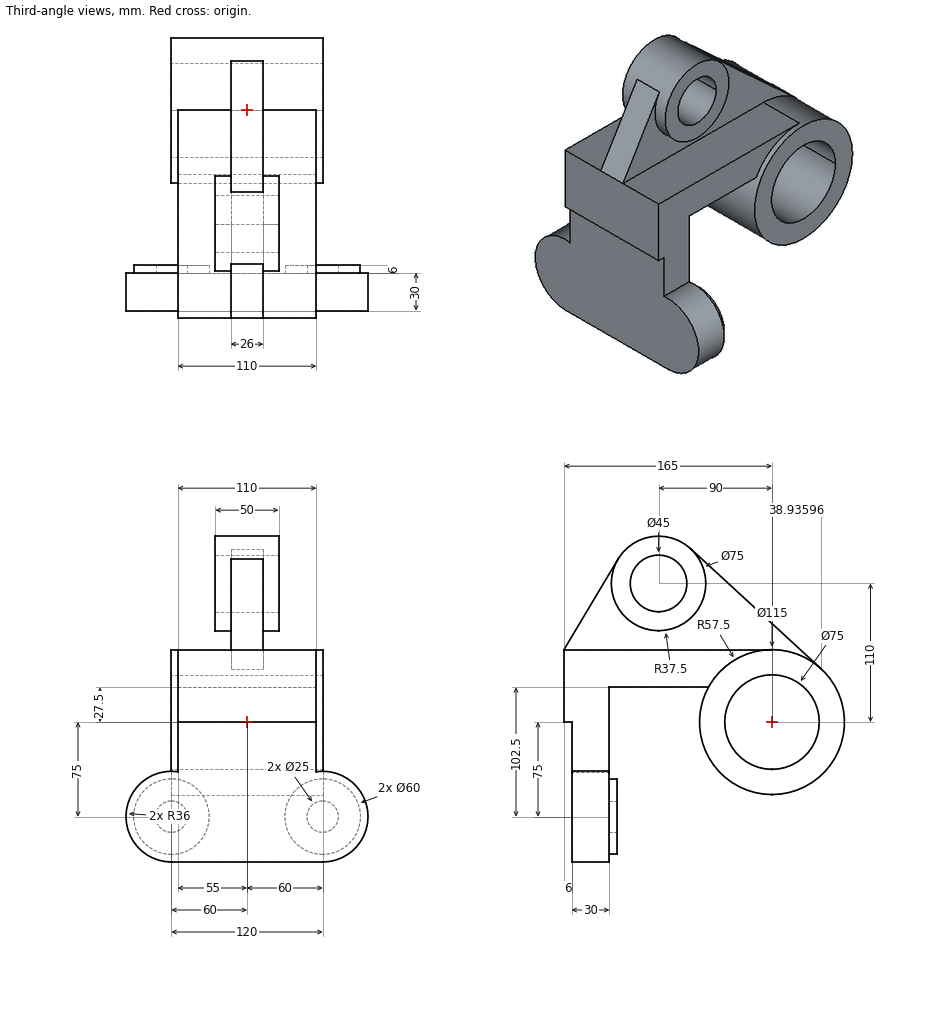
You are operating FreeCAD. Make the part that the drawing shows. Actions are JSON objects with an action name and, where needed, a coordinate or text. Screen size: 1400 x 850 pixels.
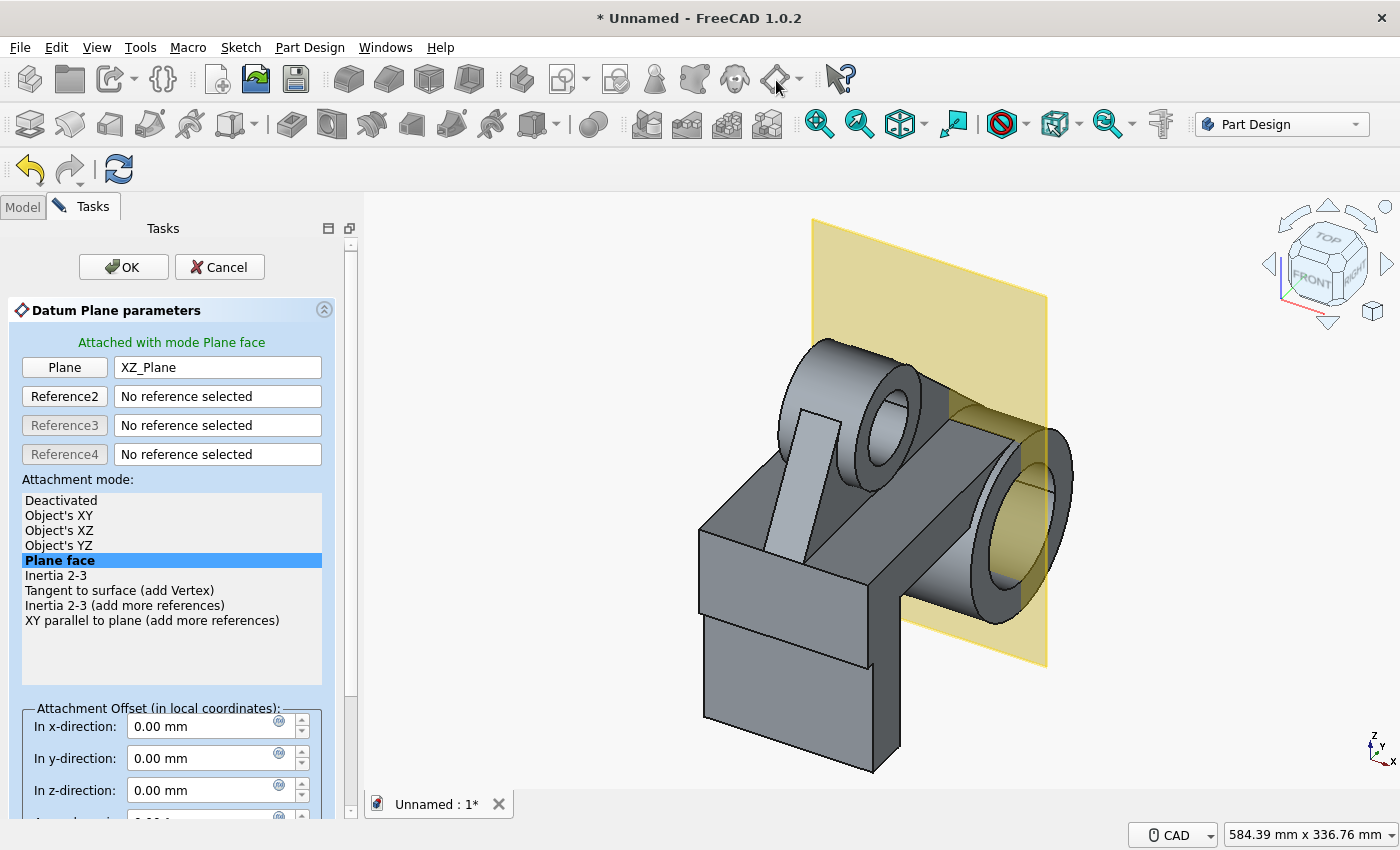
{"action": "triple_click", "coordinate": [210, 790]}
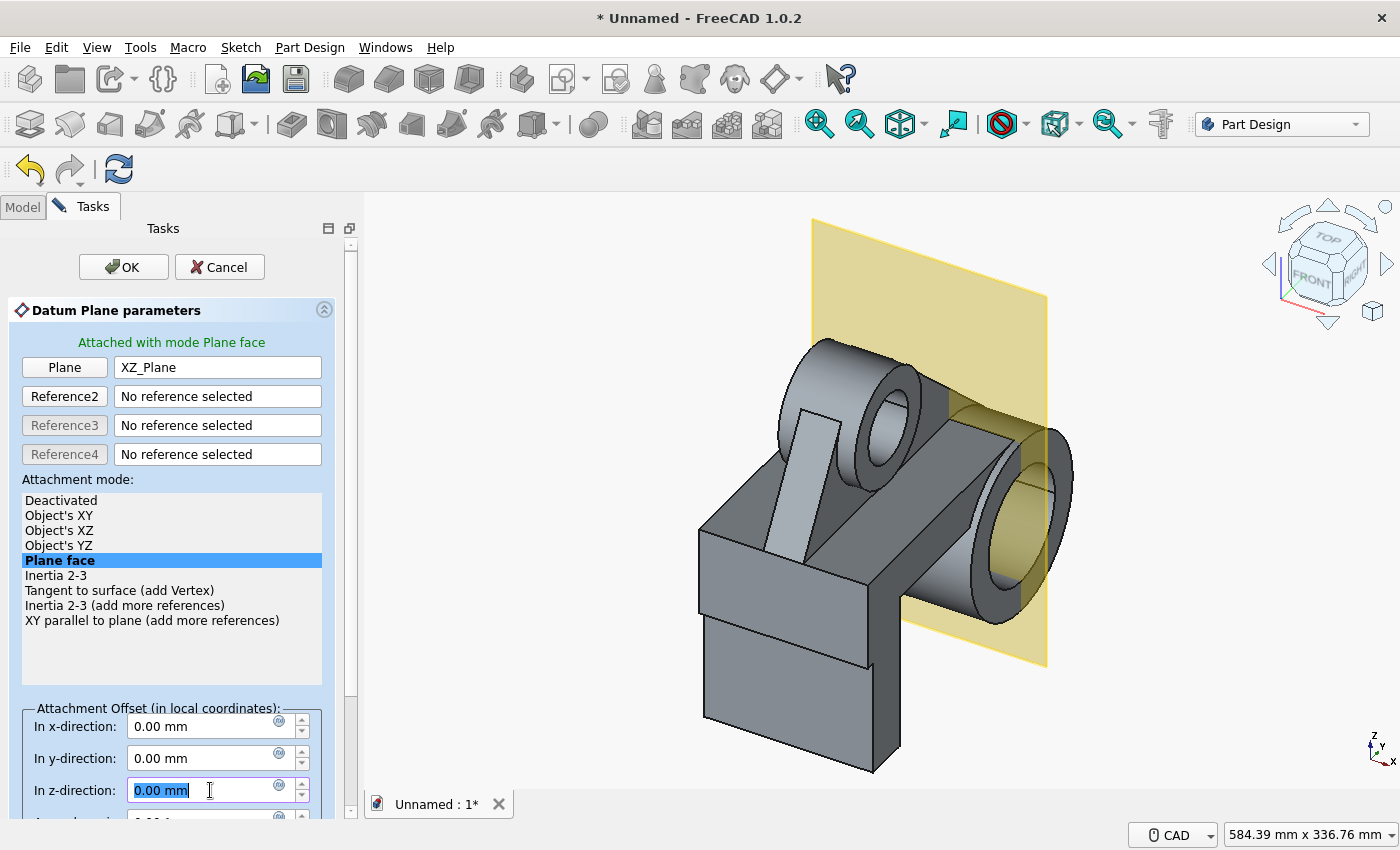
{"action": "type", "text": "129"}
{"action": "key", "text": "Tab"}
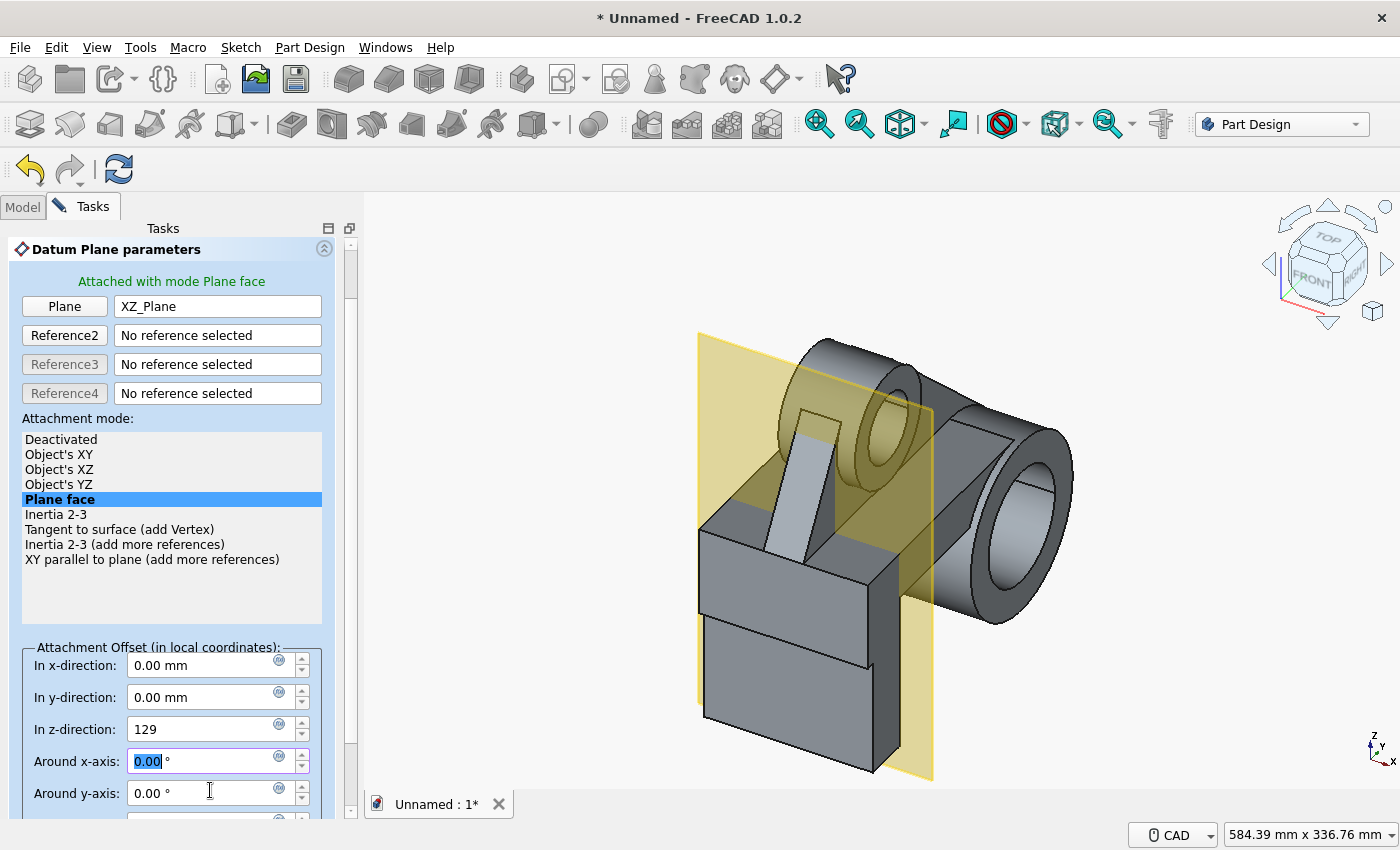
{"action": "scroll", "coordinate": [351, 528], "scroll_direction": "up", "scroll_amount": 2}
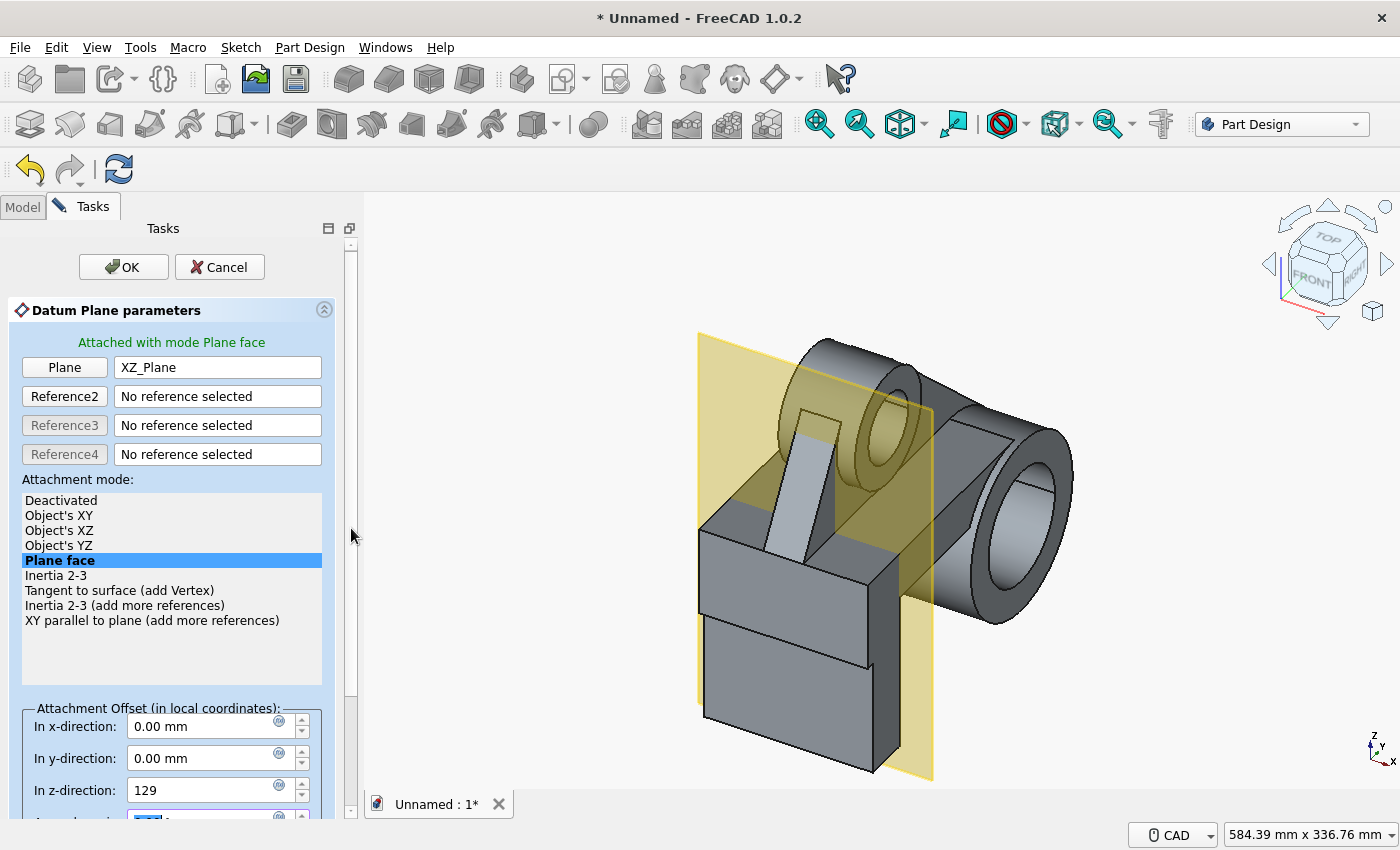
{"action": "left_click", "coordinate": [124, 267]}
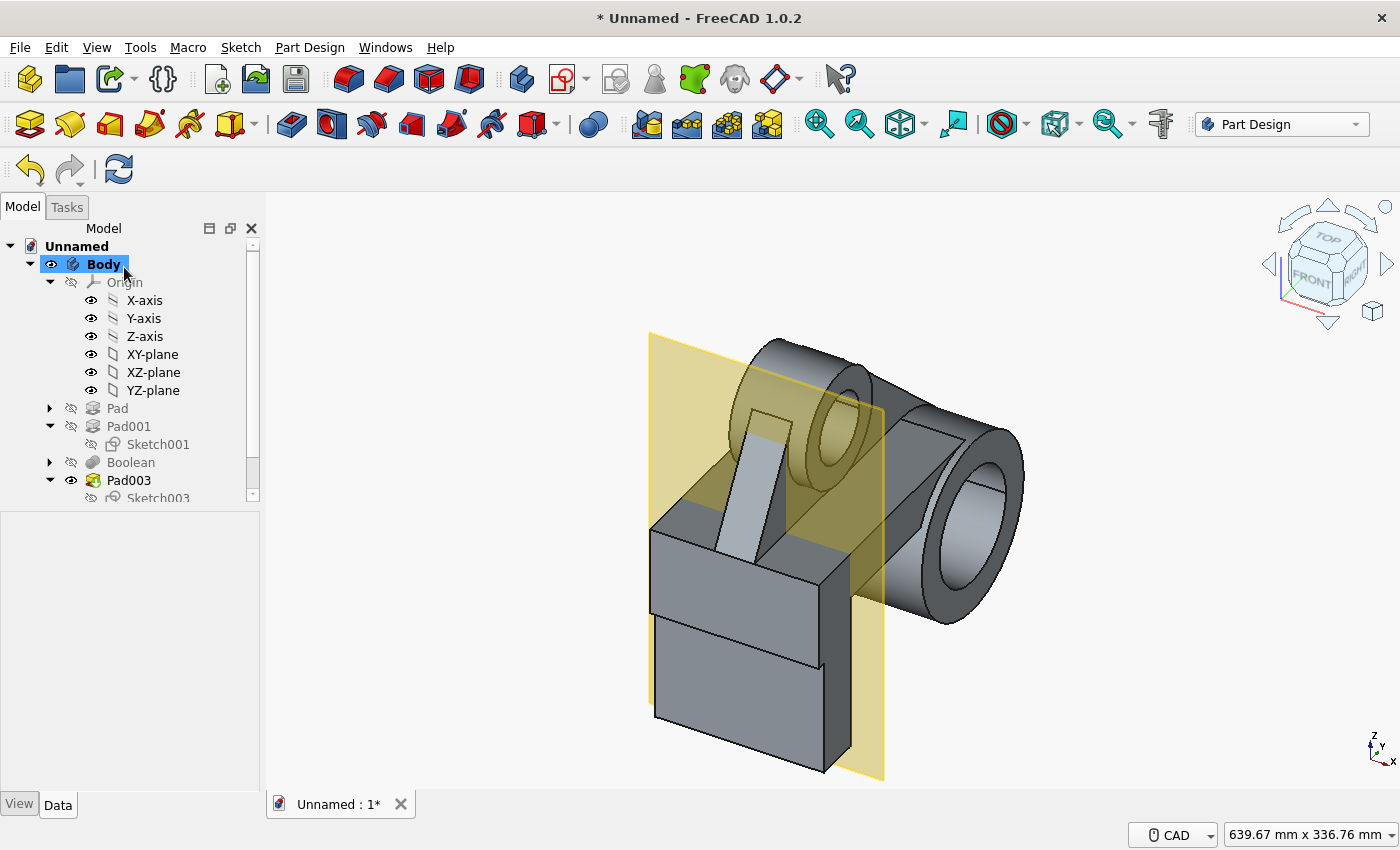
{"action": "scroll", "coordinate": [100, 368], "scroll_direction": "down", "scroll_amount": 3}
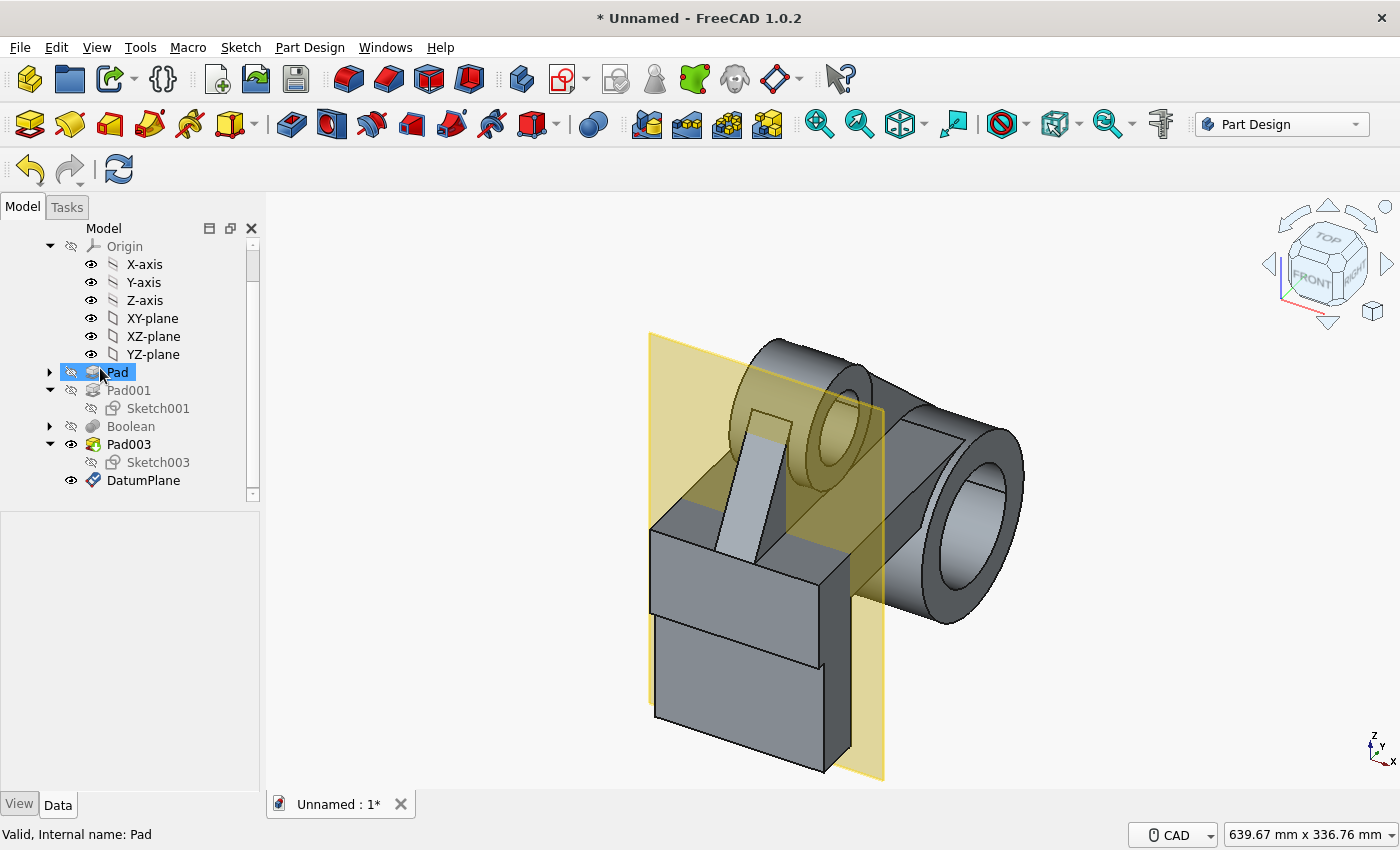
{"action": "left_click", "coordinate": [116, 480]}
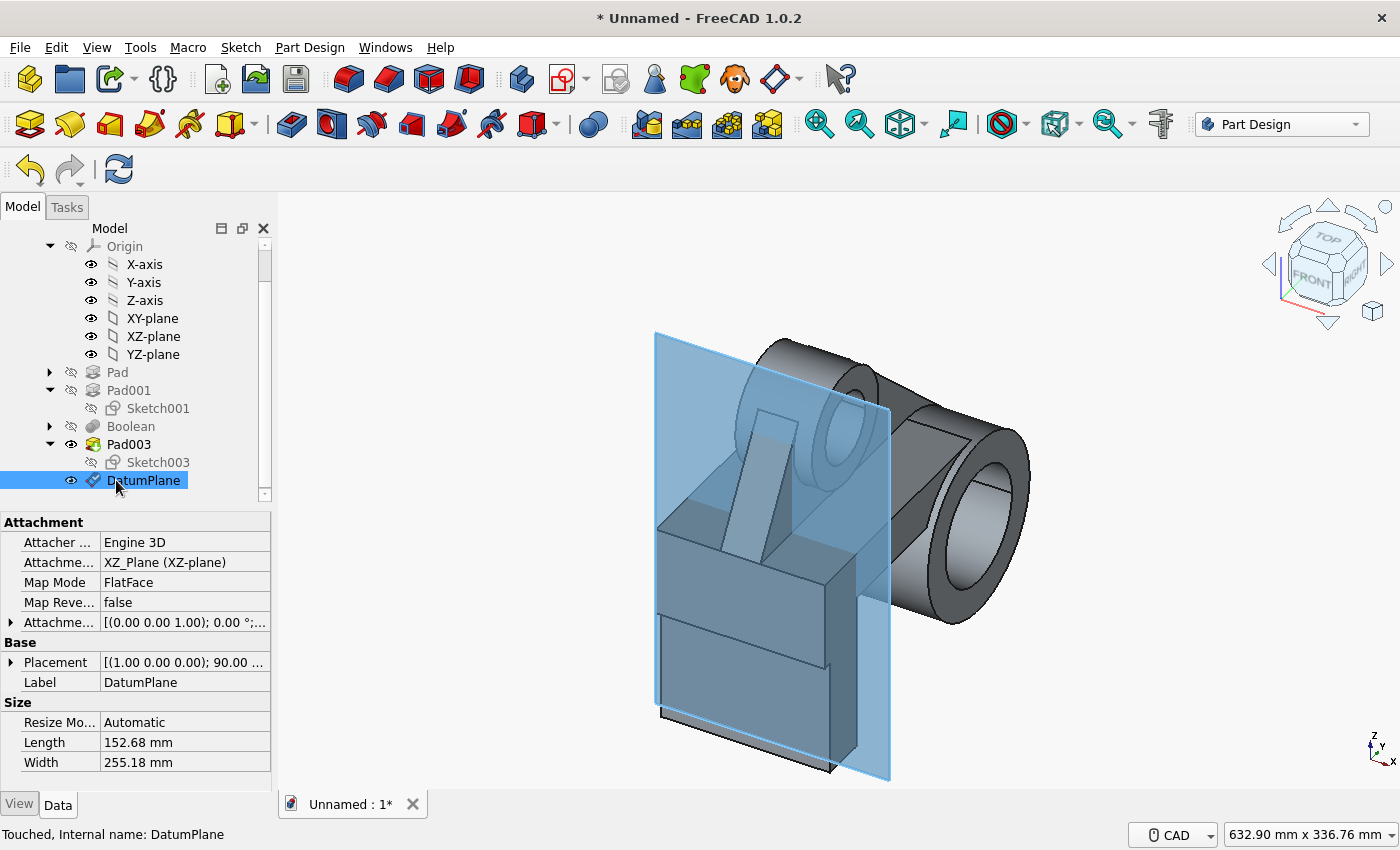
{"action": "left_click", "coordinate": [562, 80]}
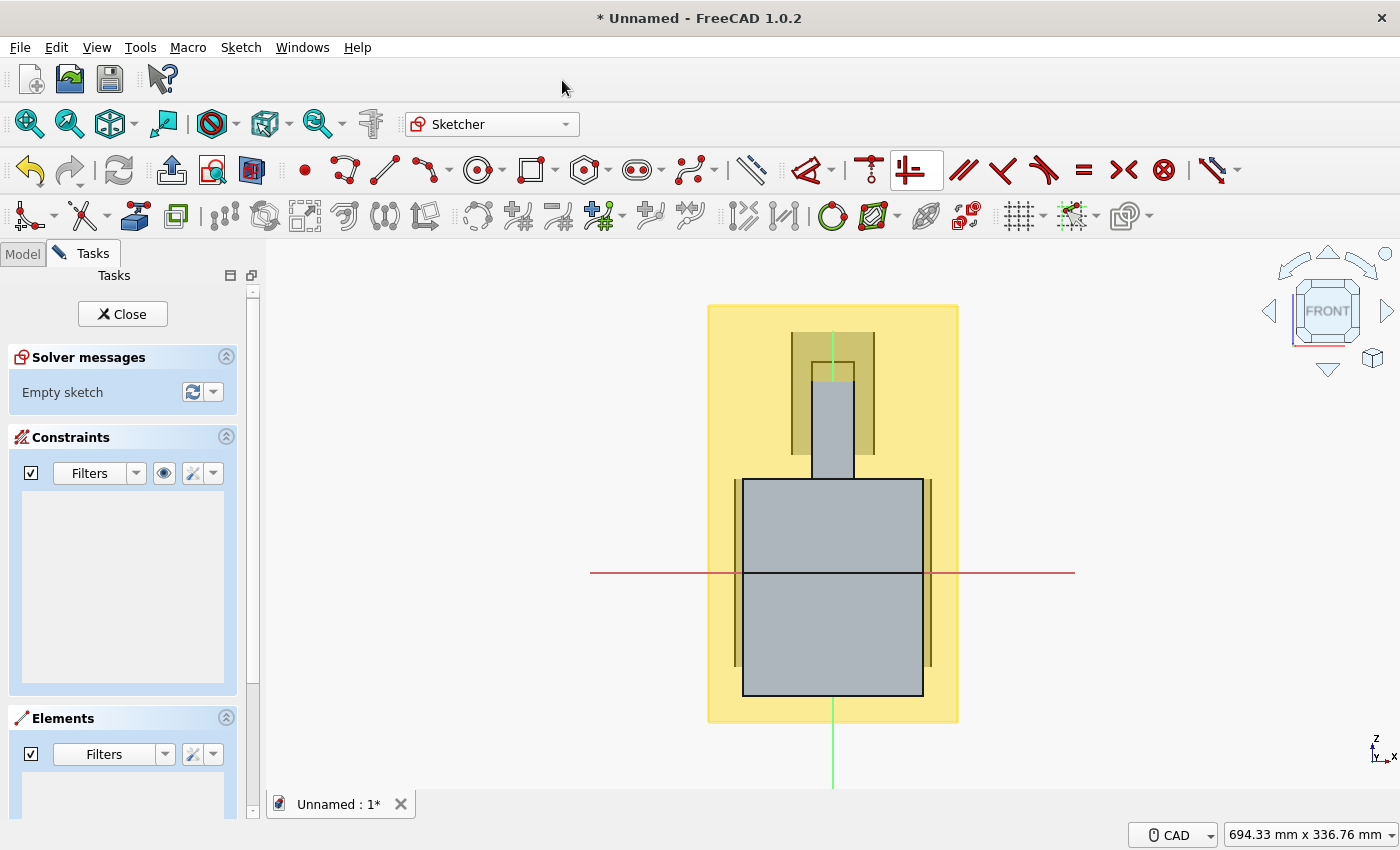
{"action": "left_click", "coordinate": [252, 170]}